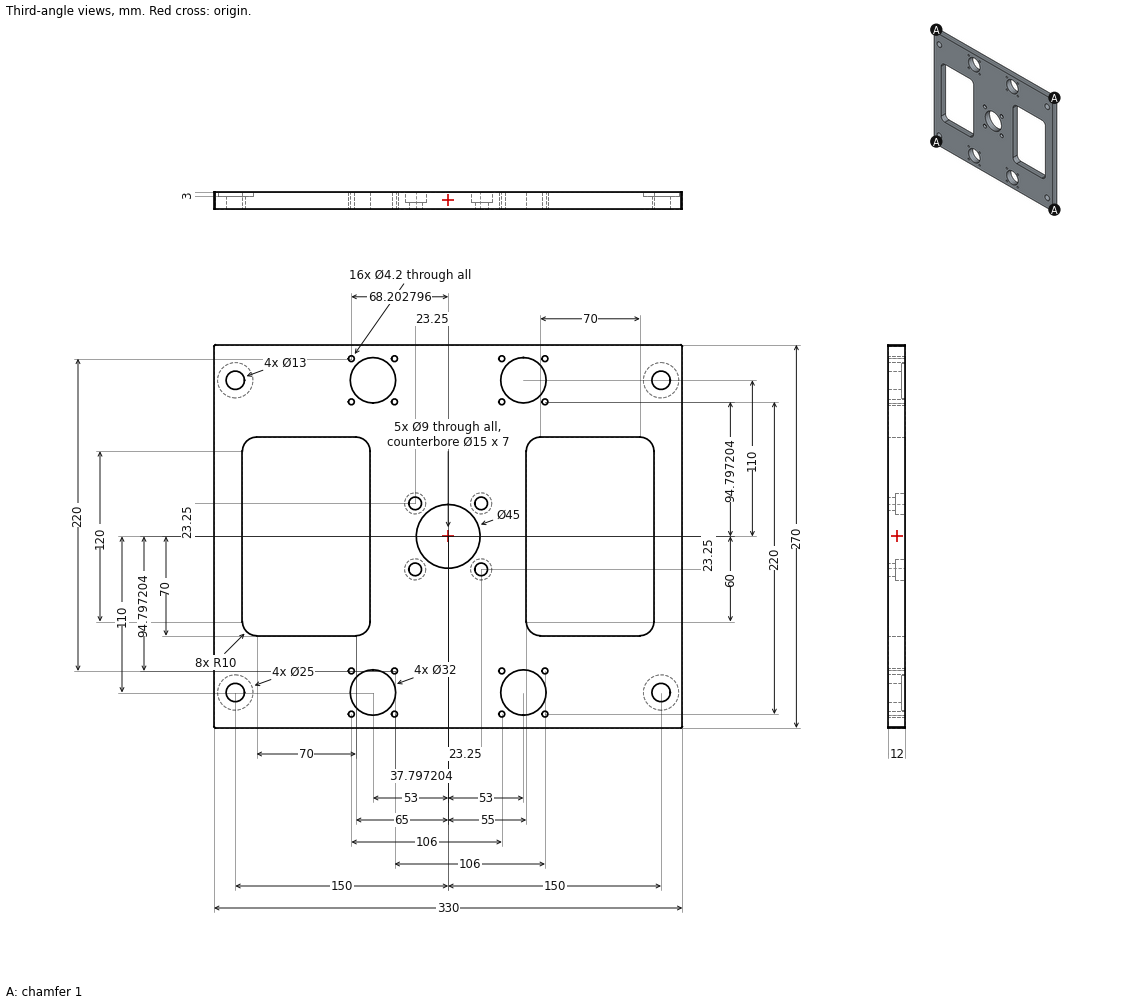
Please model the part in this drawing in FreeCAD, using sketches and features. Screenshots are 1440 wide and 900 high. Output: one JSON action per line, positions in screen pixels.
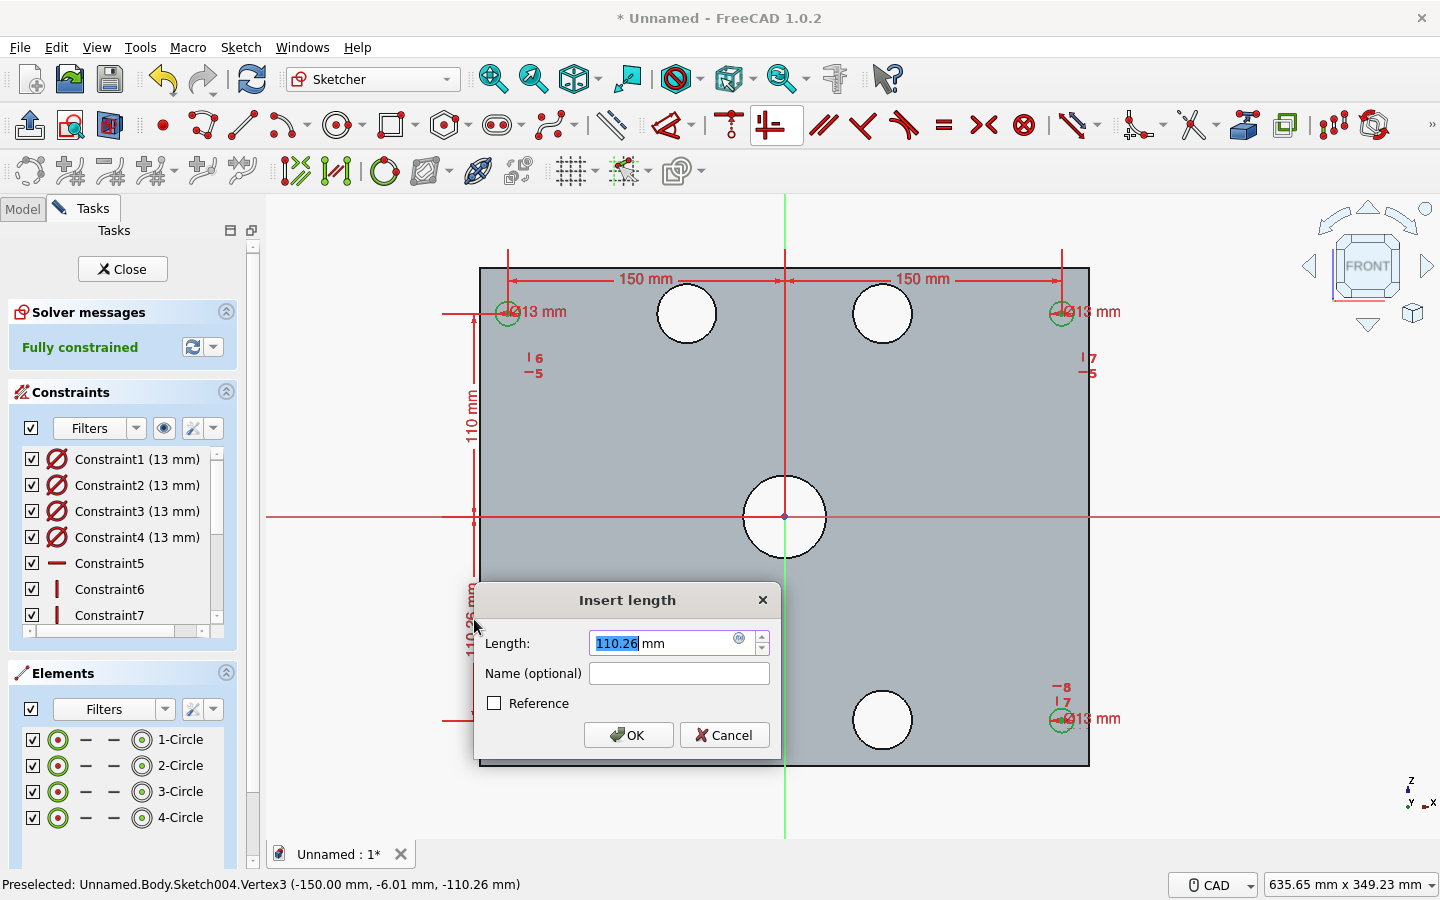
{"action": "type", "text": "110"}
{"action": "key", "text": "Return"}
{"action": "key", "text": "Escape"}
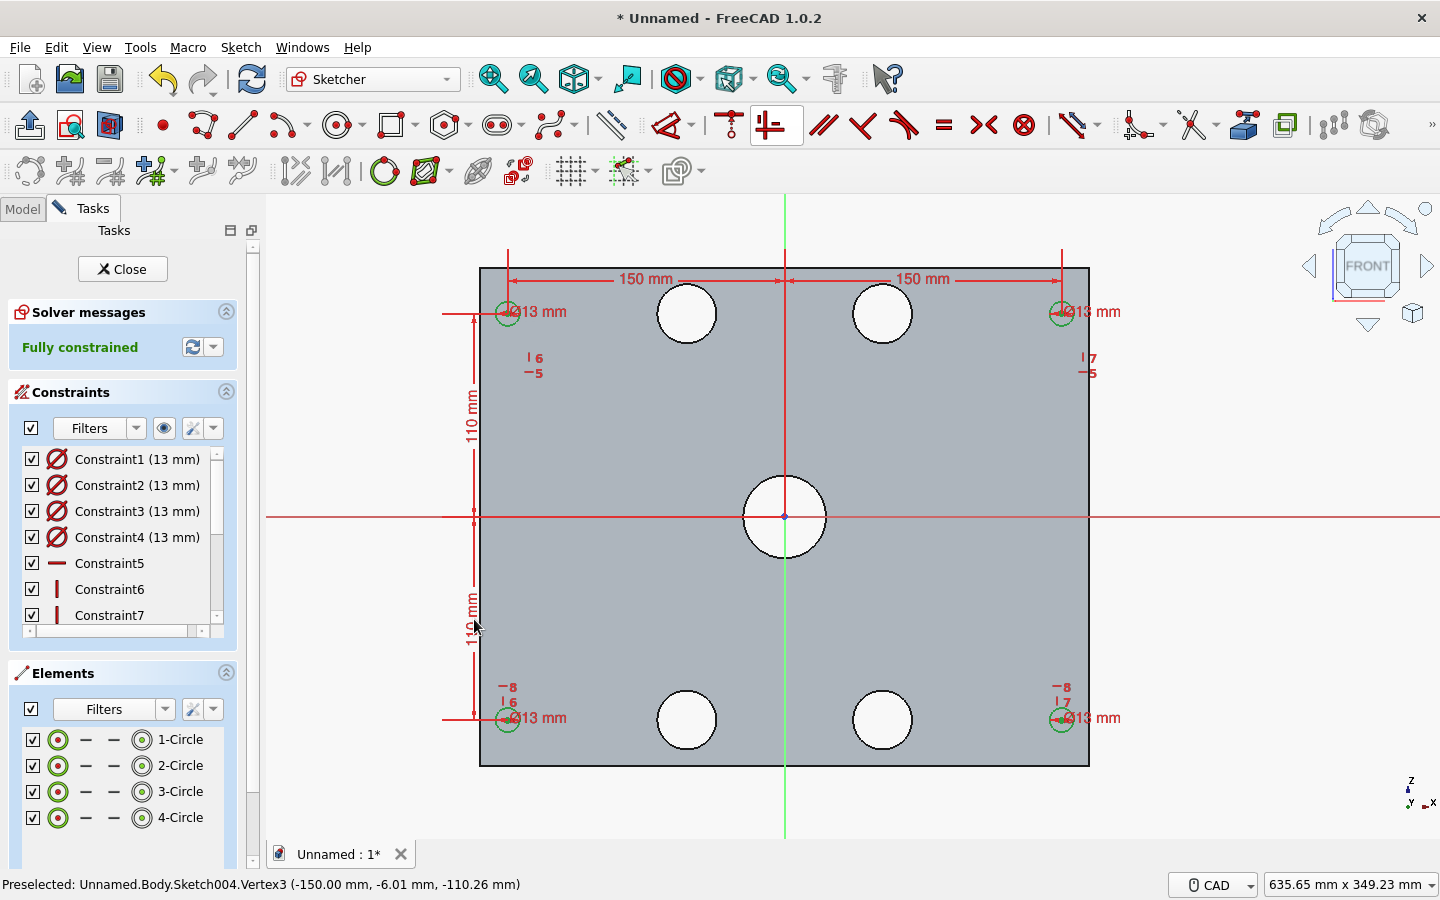
{"action": "left_click", "coordinate": [123, 269]}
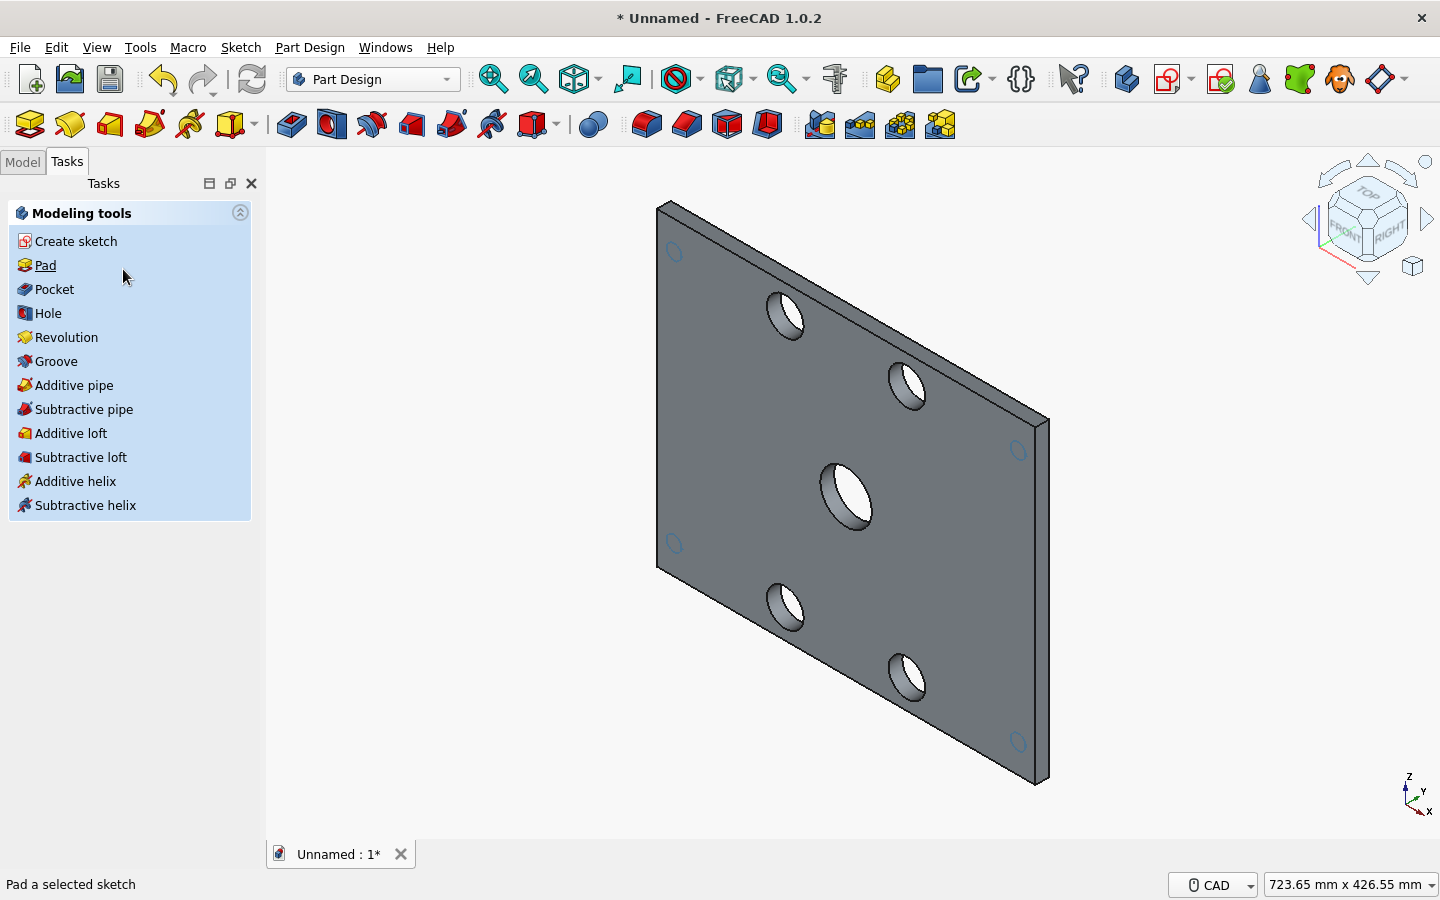
{"action": "left_click", "coordinate": [292, 124]}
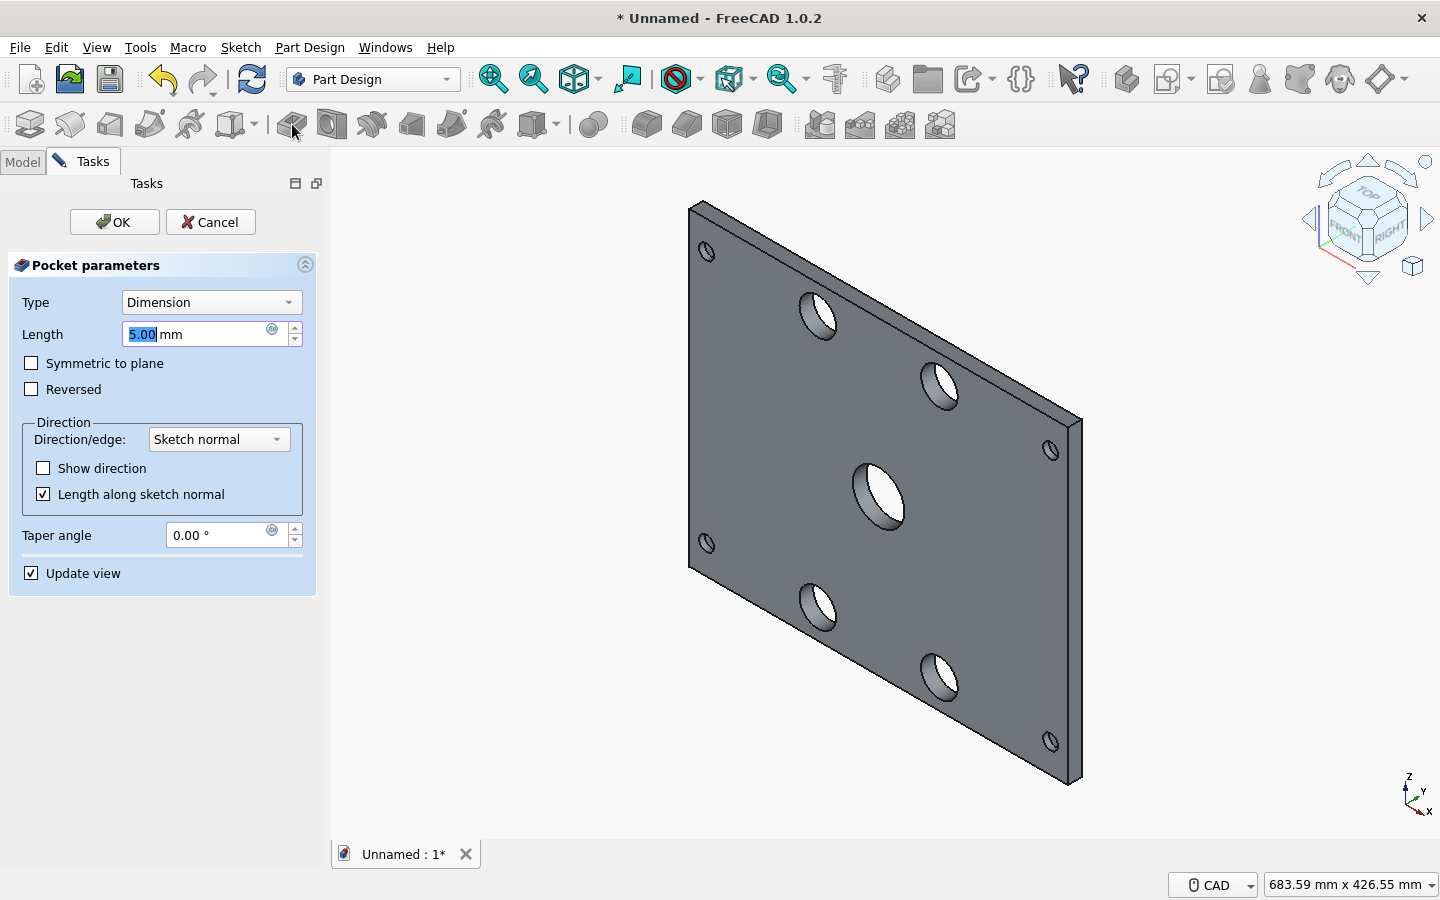
{"action": "left_click", "coordinate": [212, 302]}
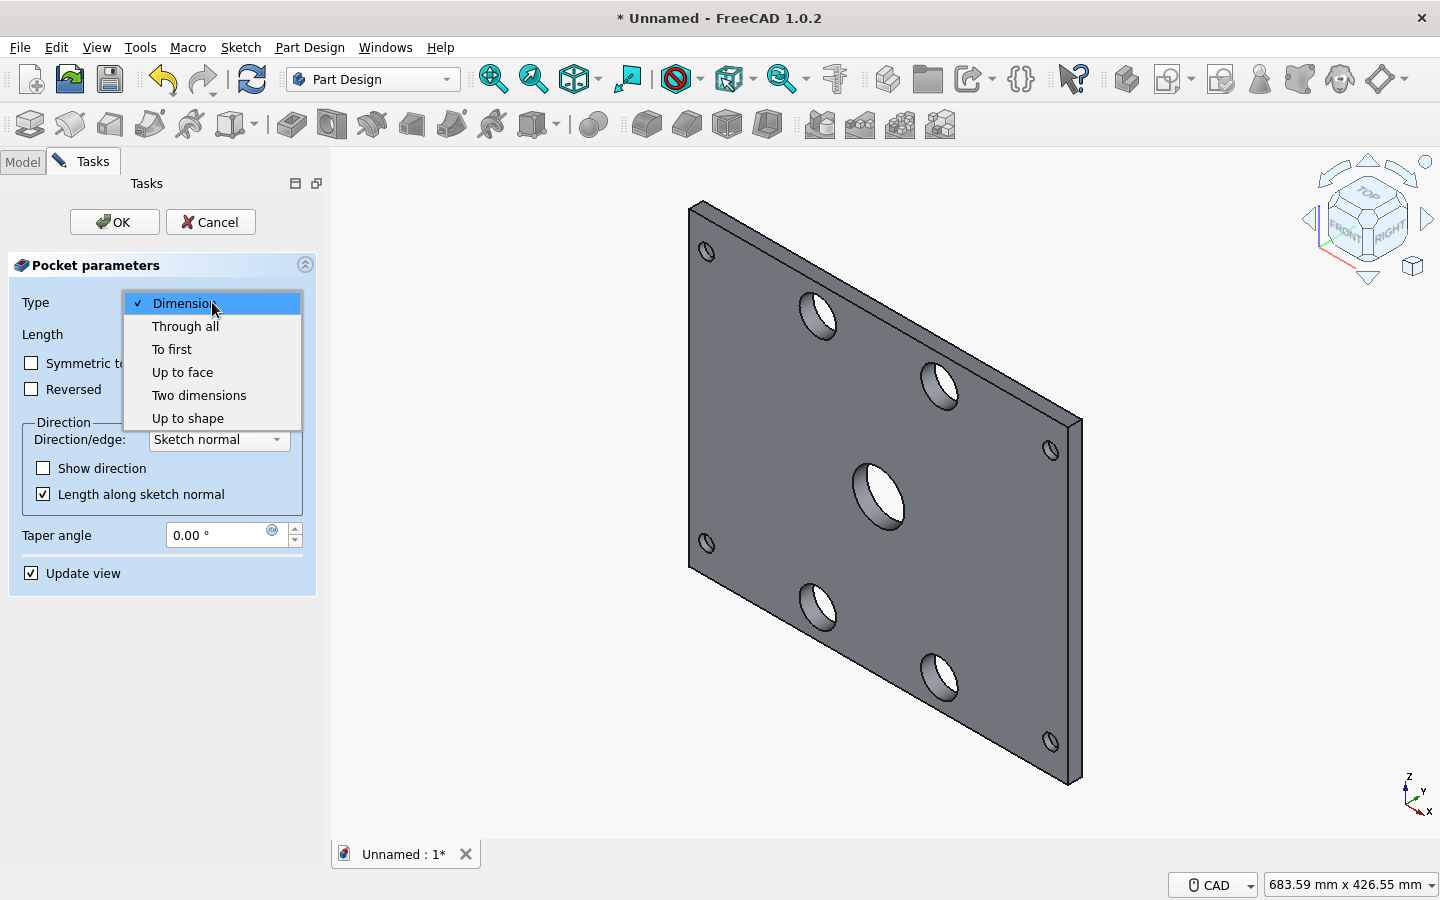
{"action": "left_click", "coordinate": [212, 326]}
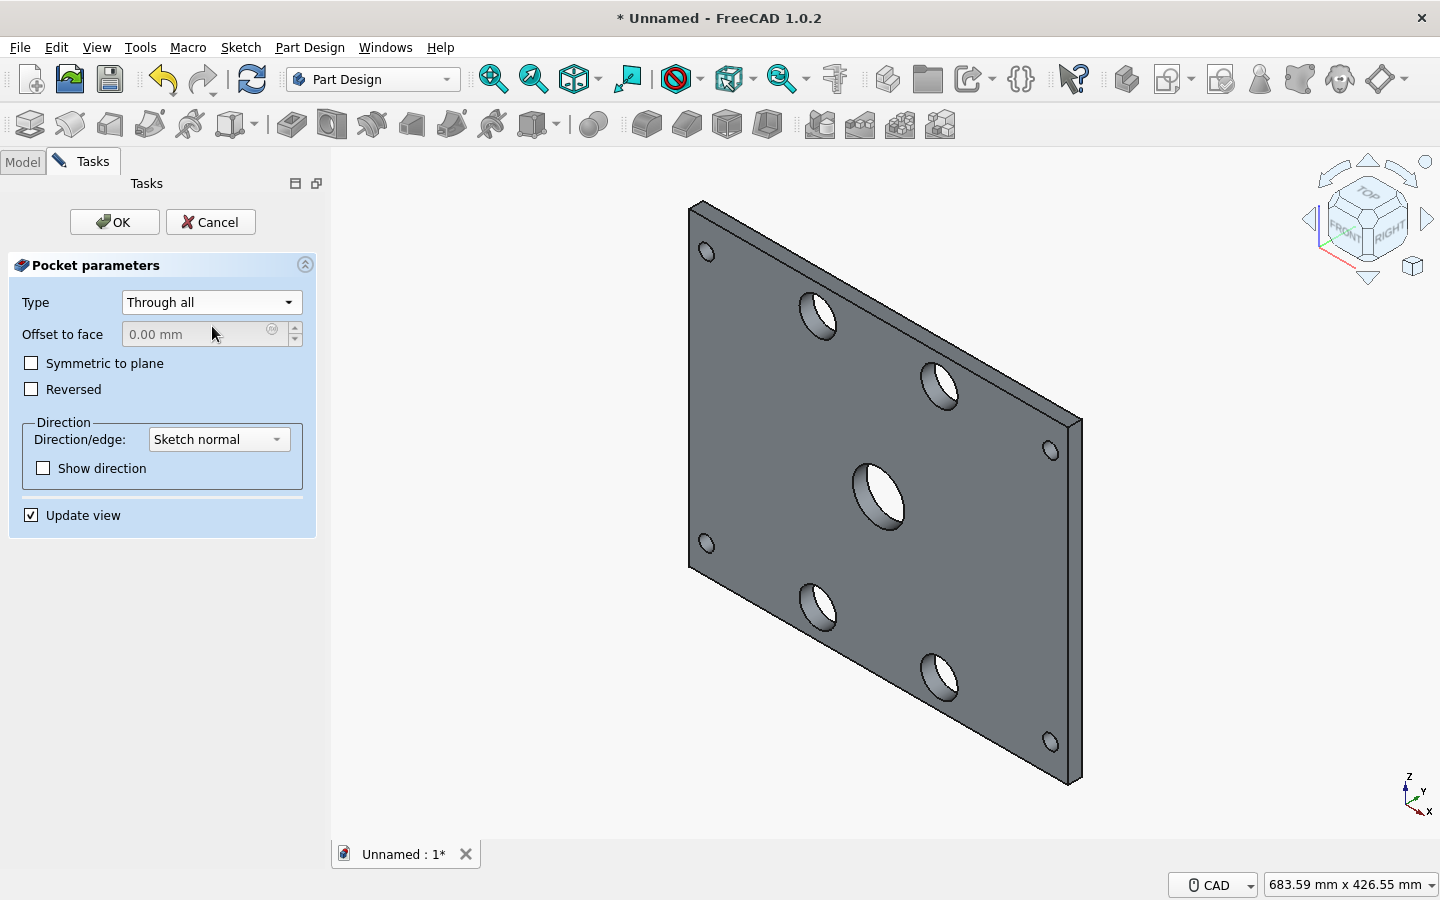
{"action": "left_click", "coordinate": [115, 222]}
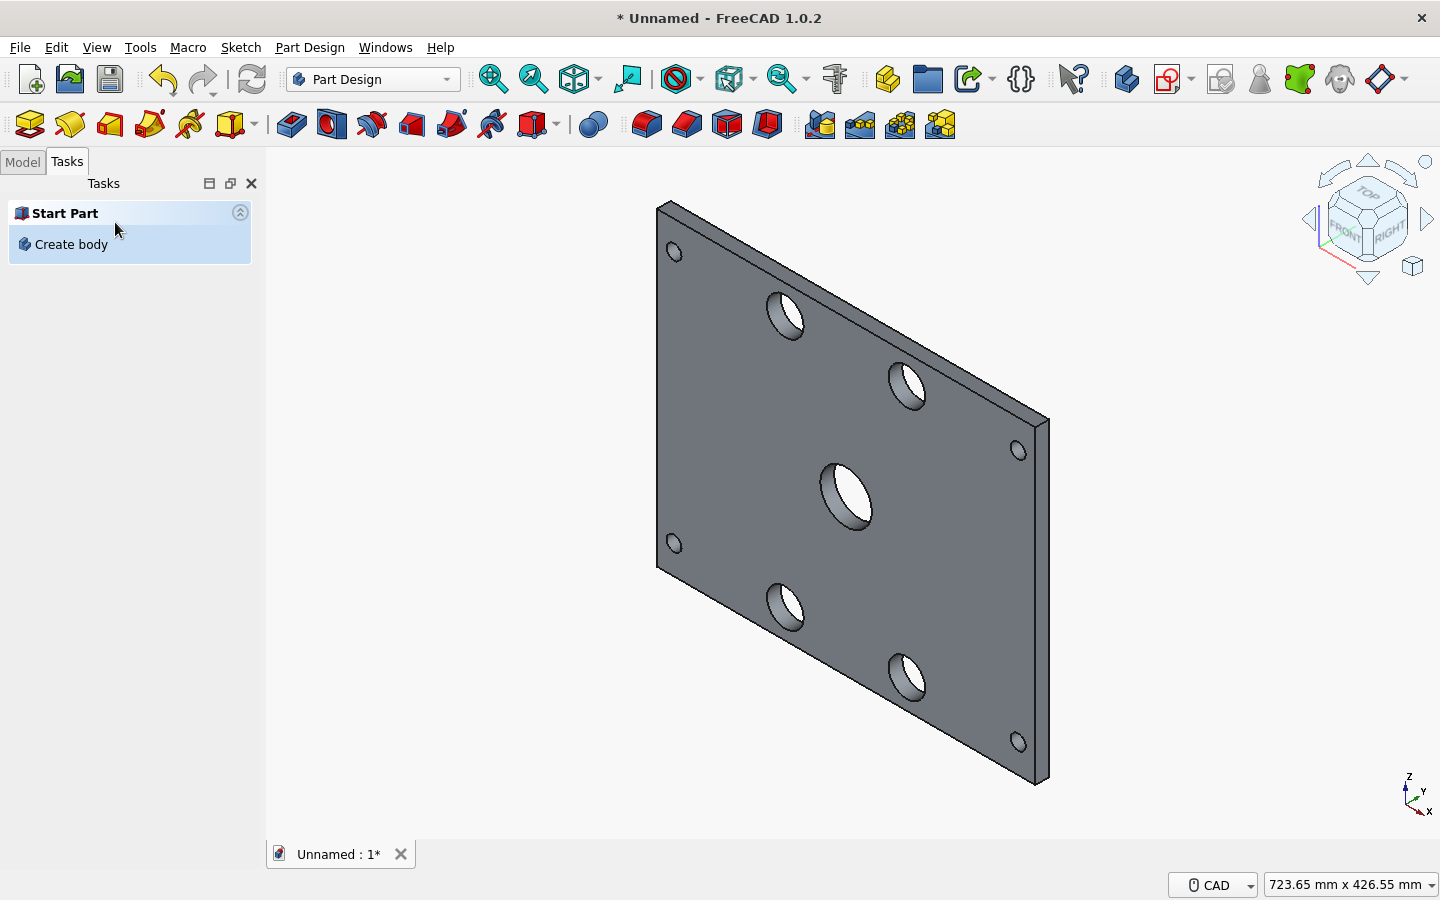
{"action": "key", "text": "4"}